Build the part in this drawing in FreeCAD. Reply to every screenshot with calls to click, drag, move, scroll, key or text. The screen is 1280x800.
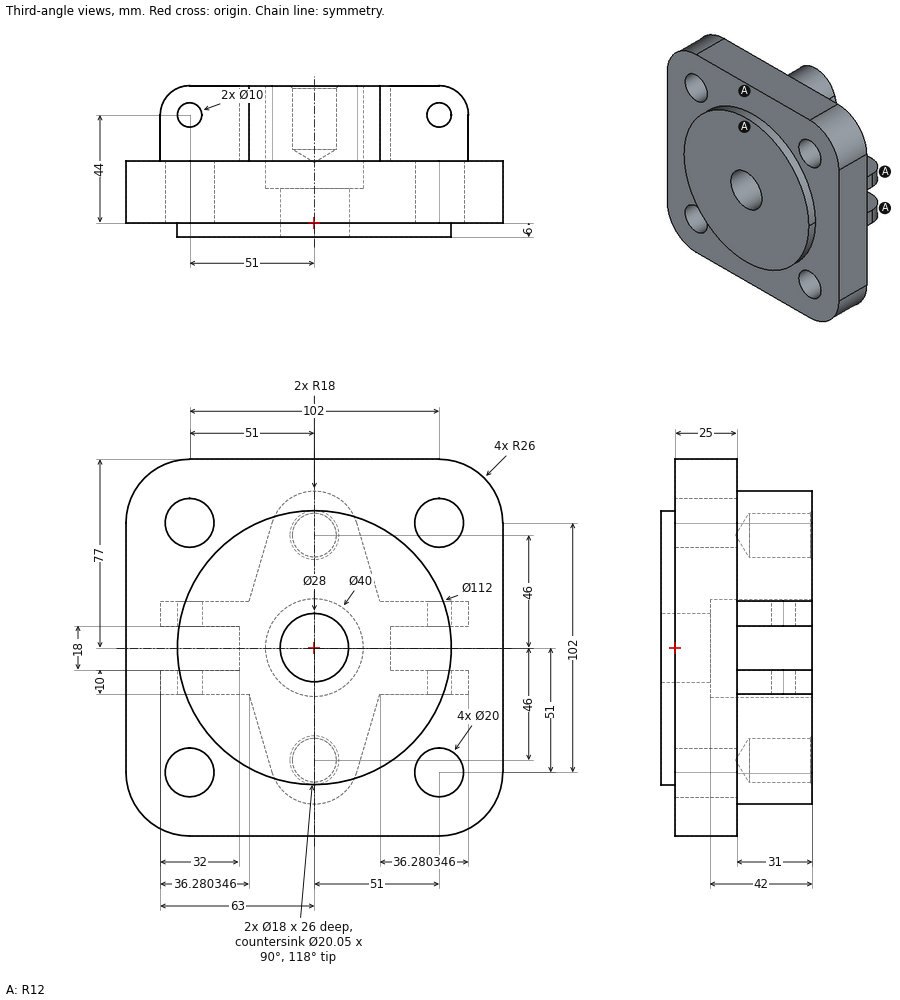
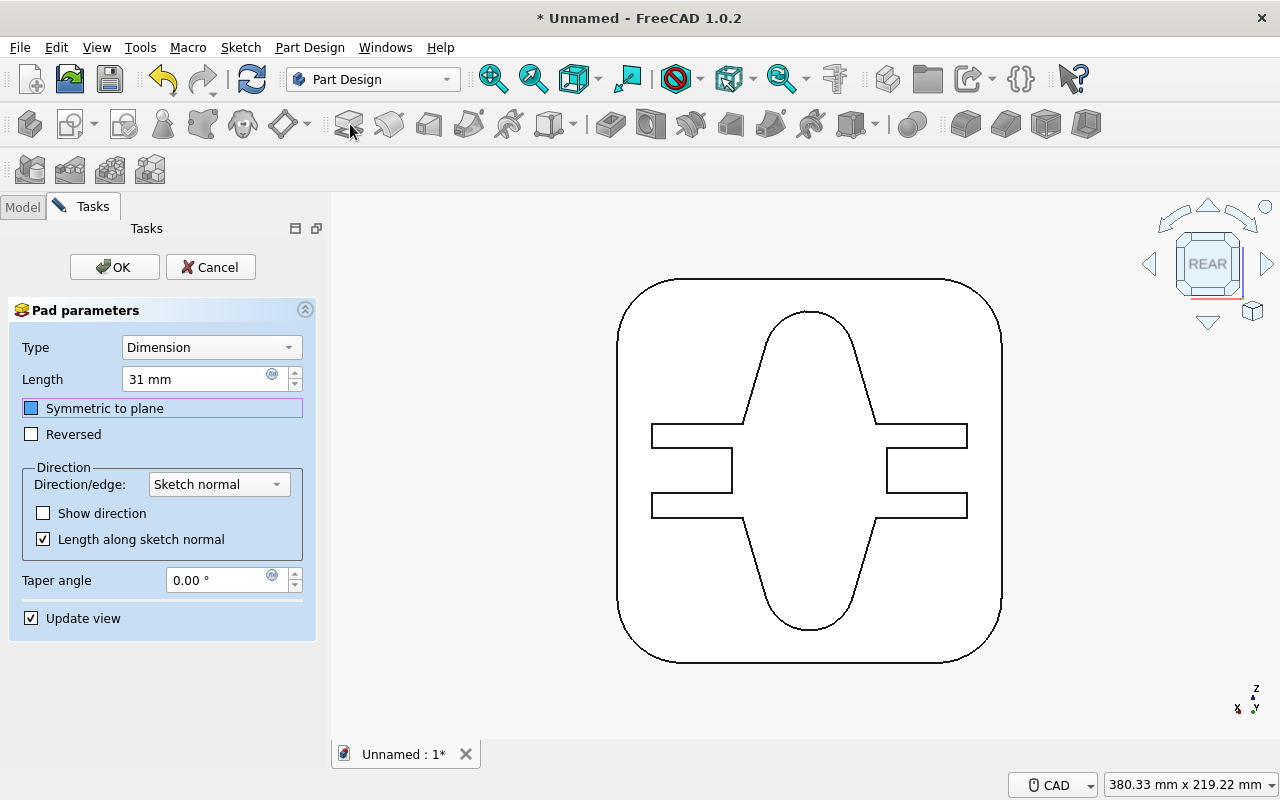
click(115, 267)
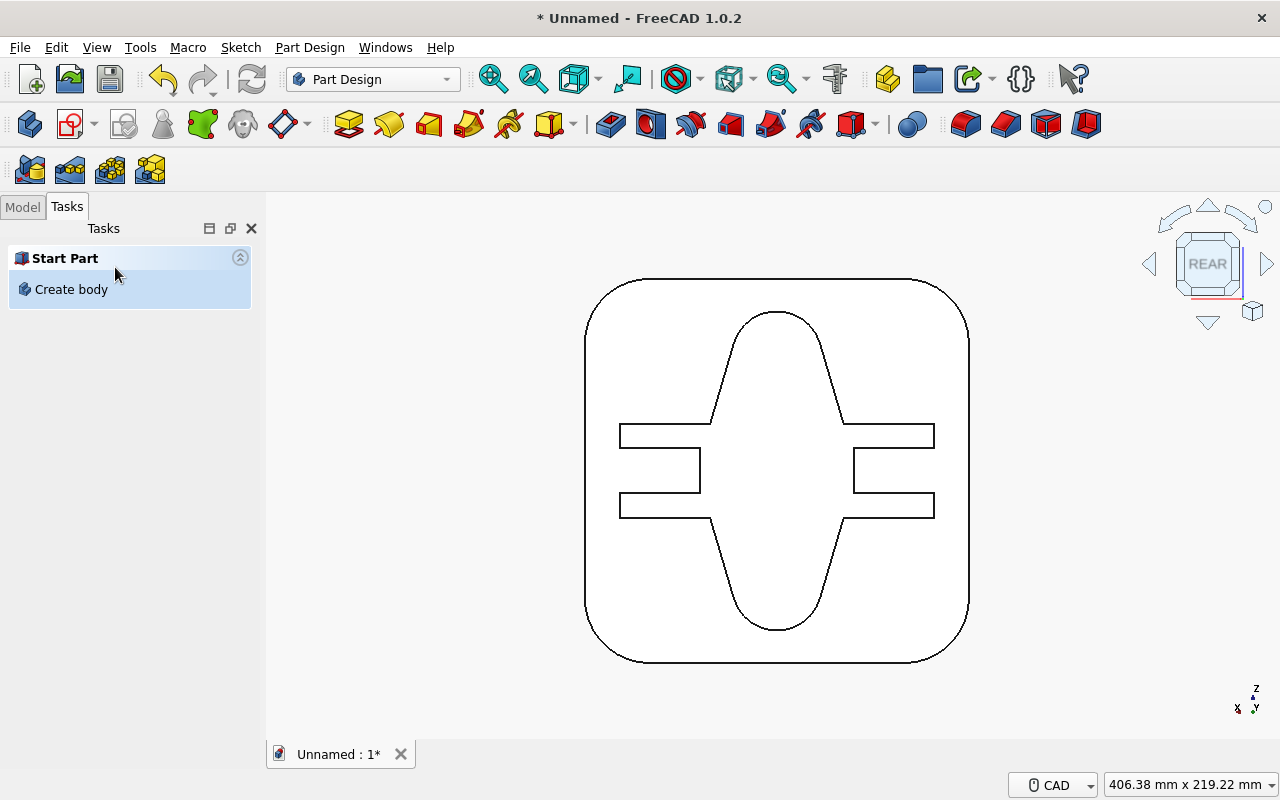
click(934, 435)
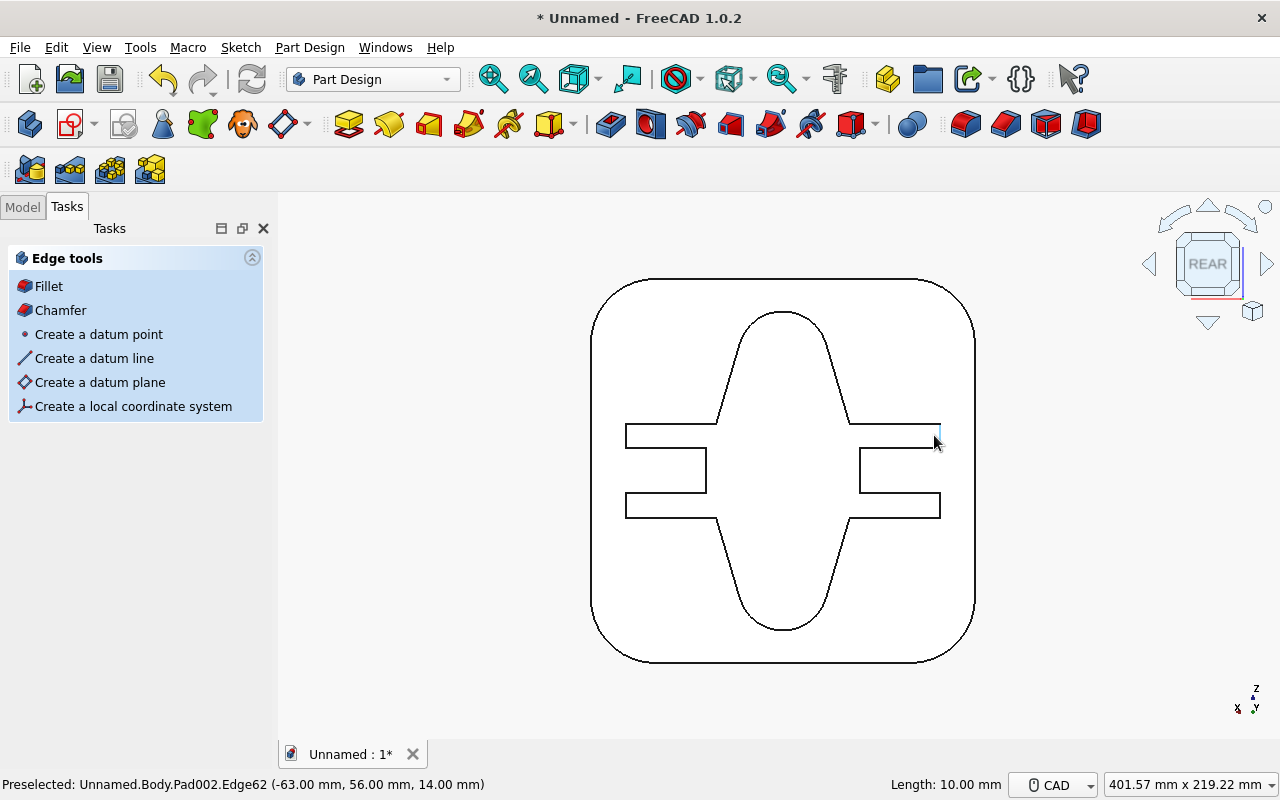
click(940, 505, ctrl)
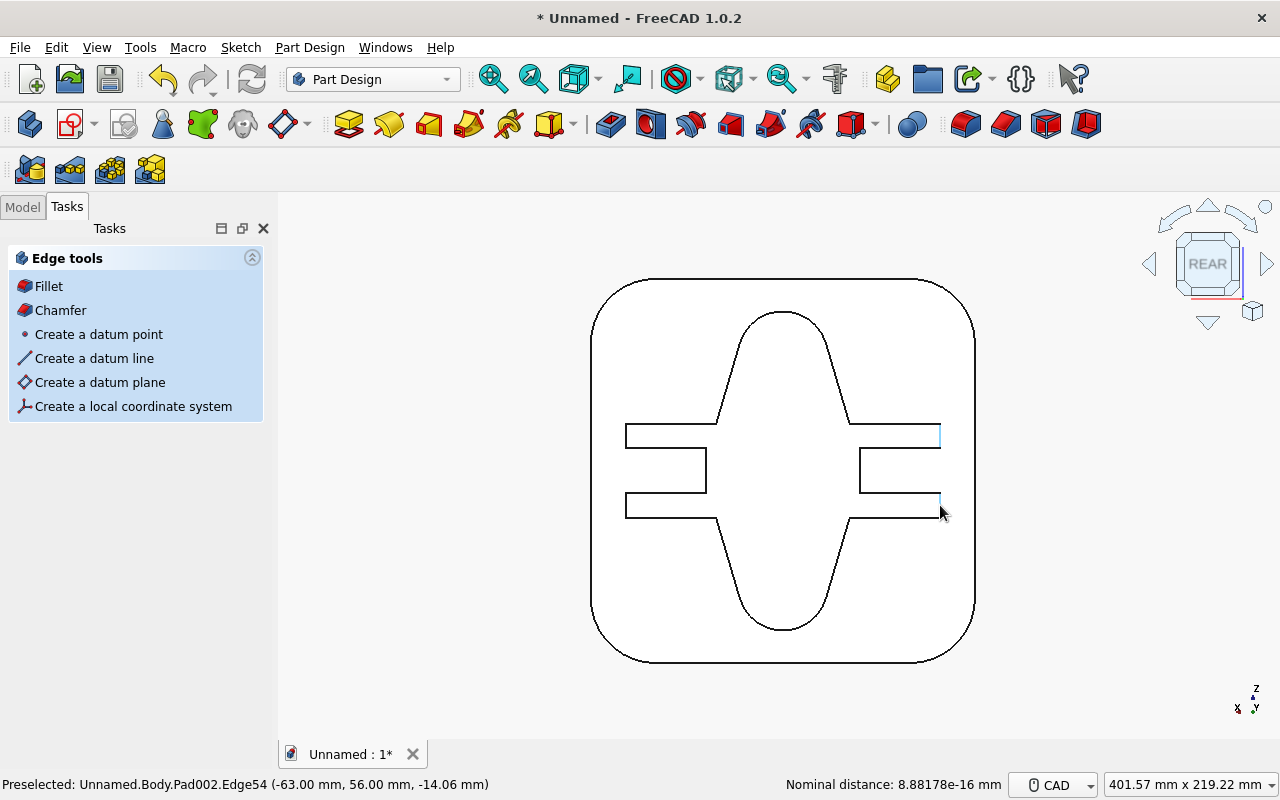
key(0)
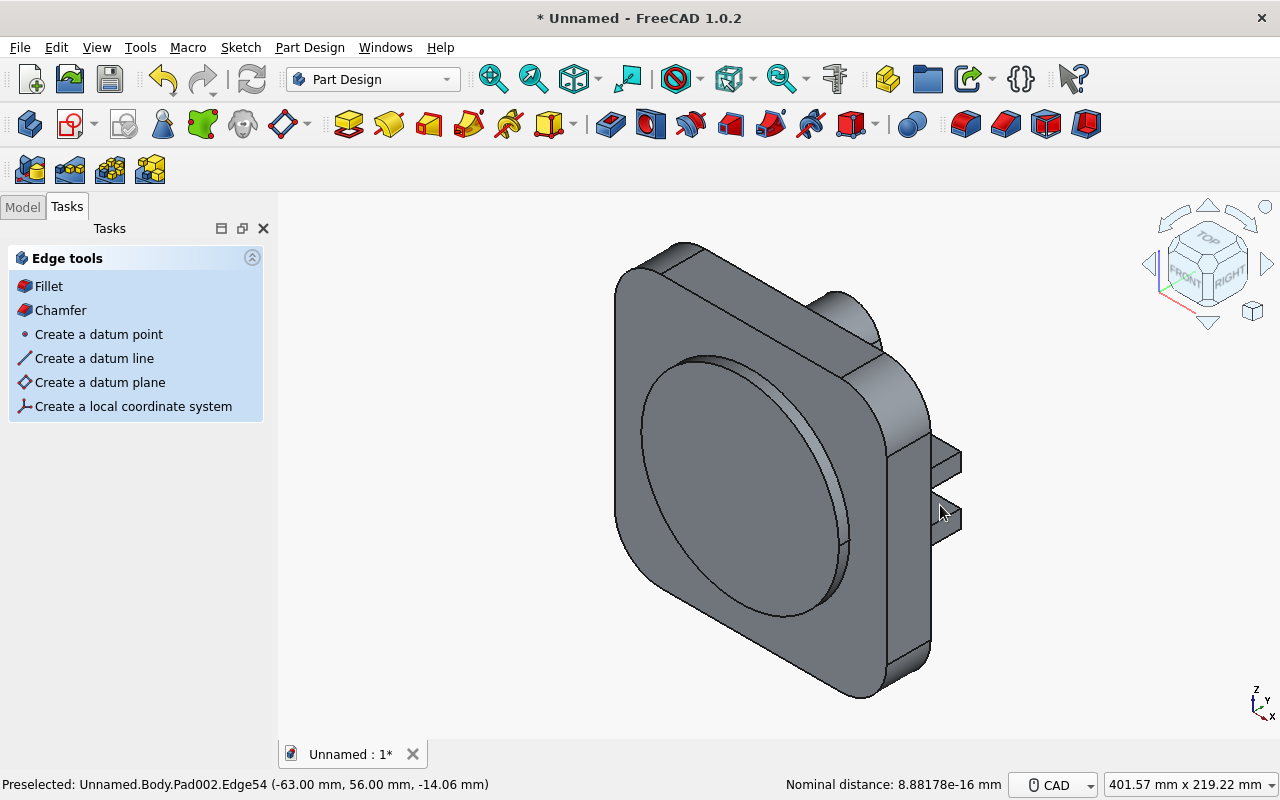
key(v)
key(f)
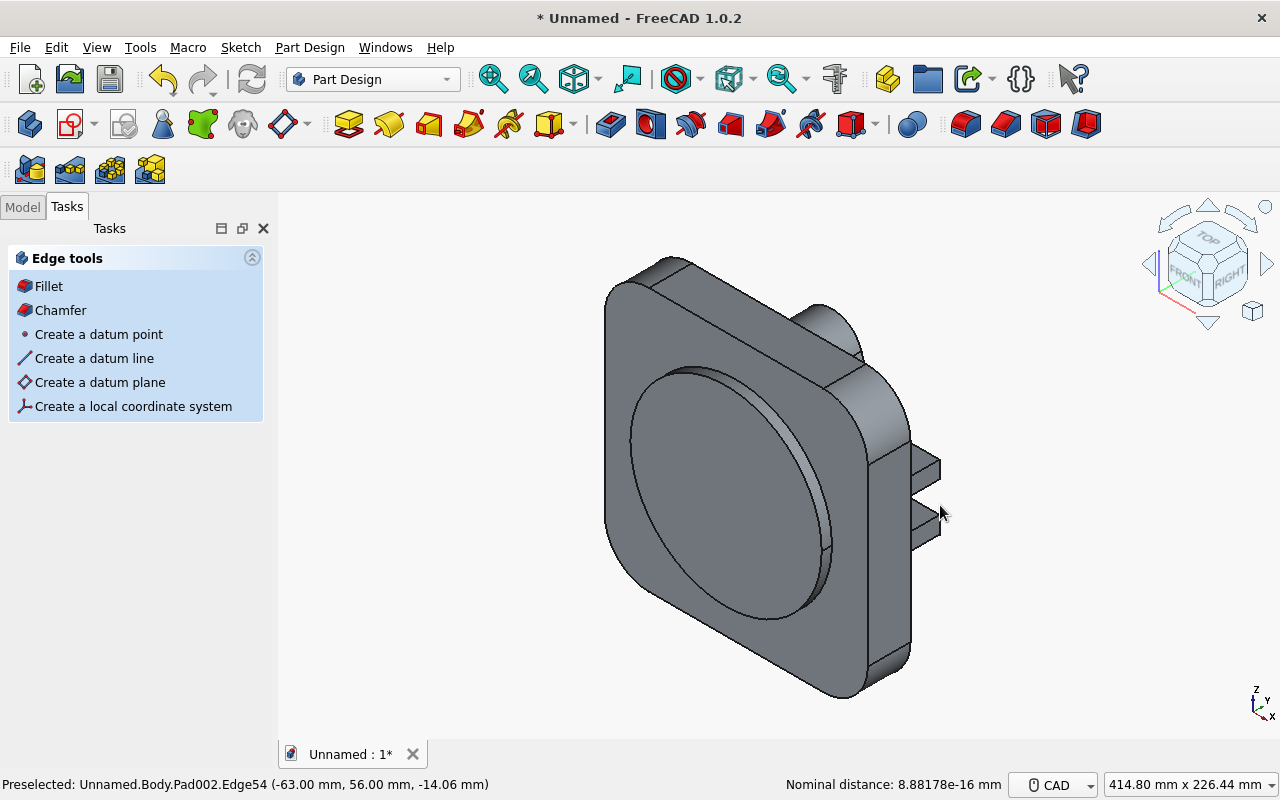
key(2)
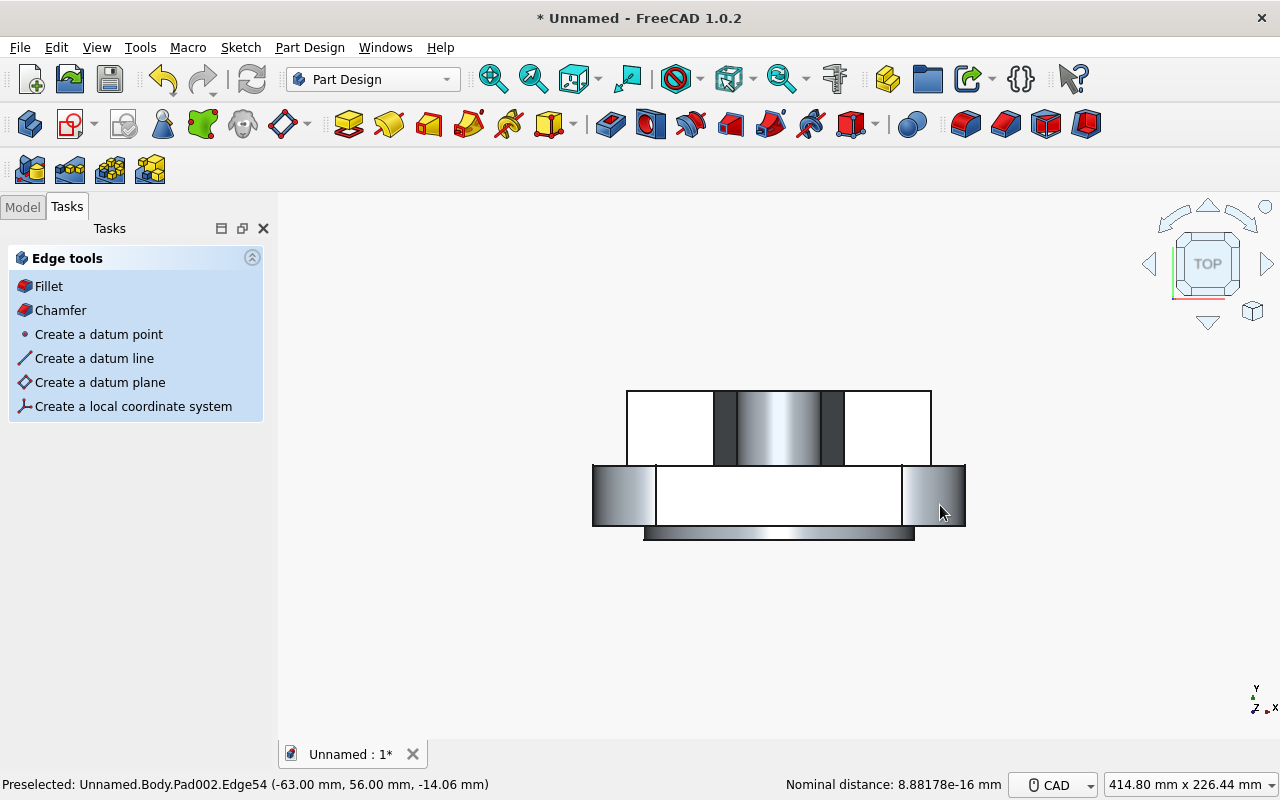
click(494, 80)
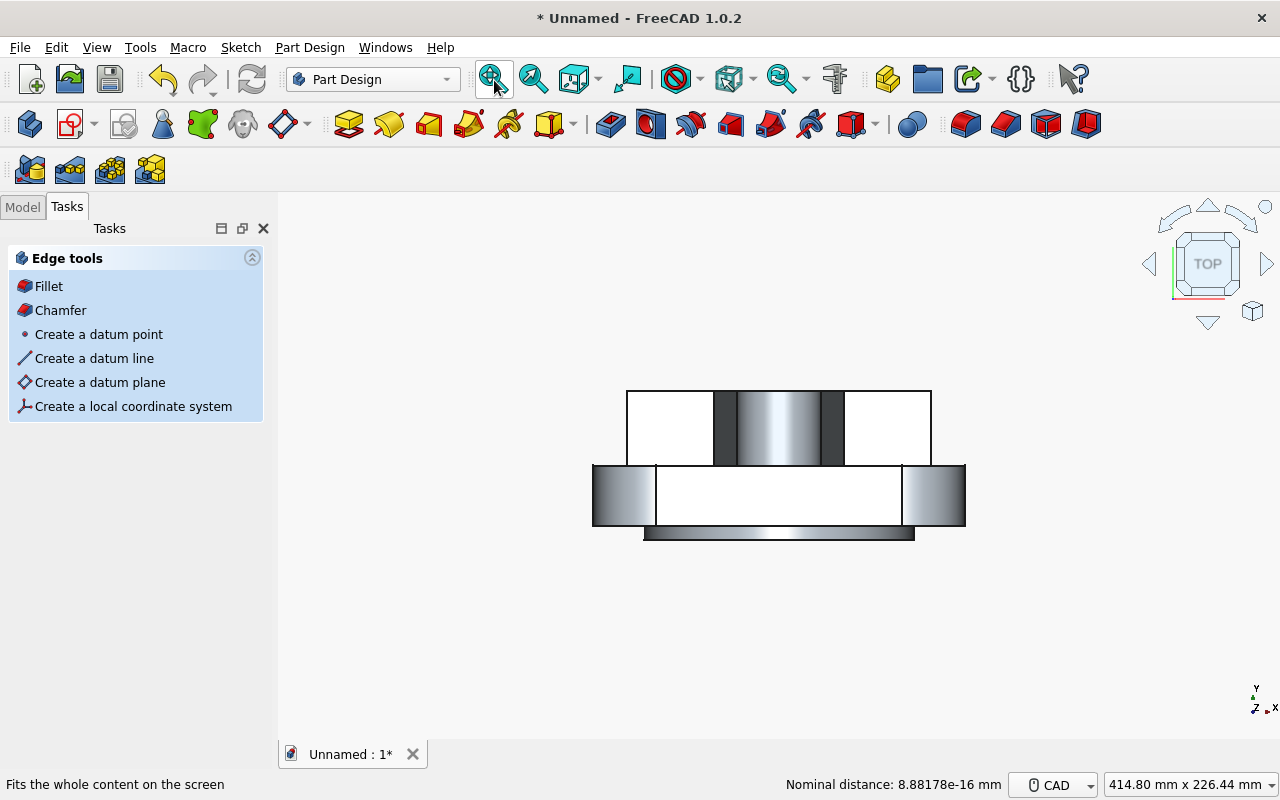
key(1)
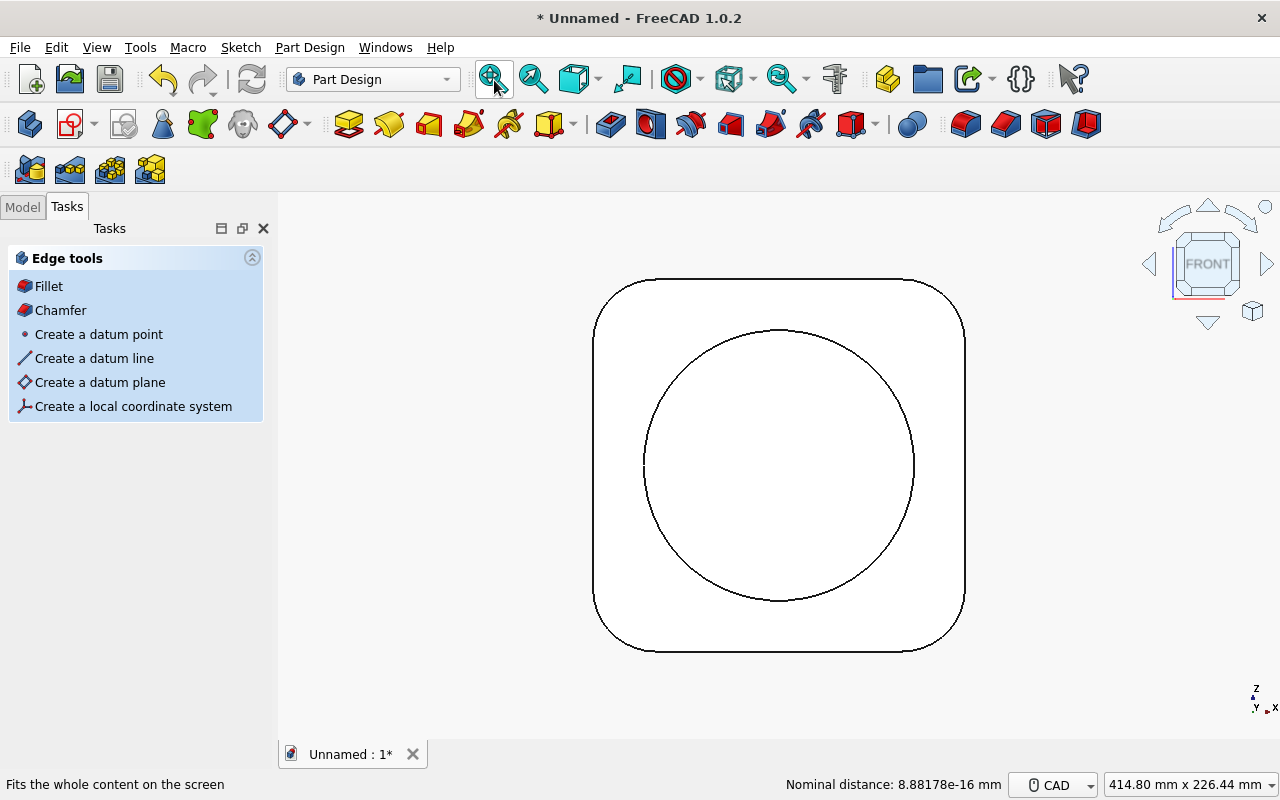
key(3)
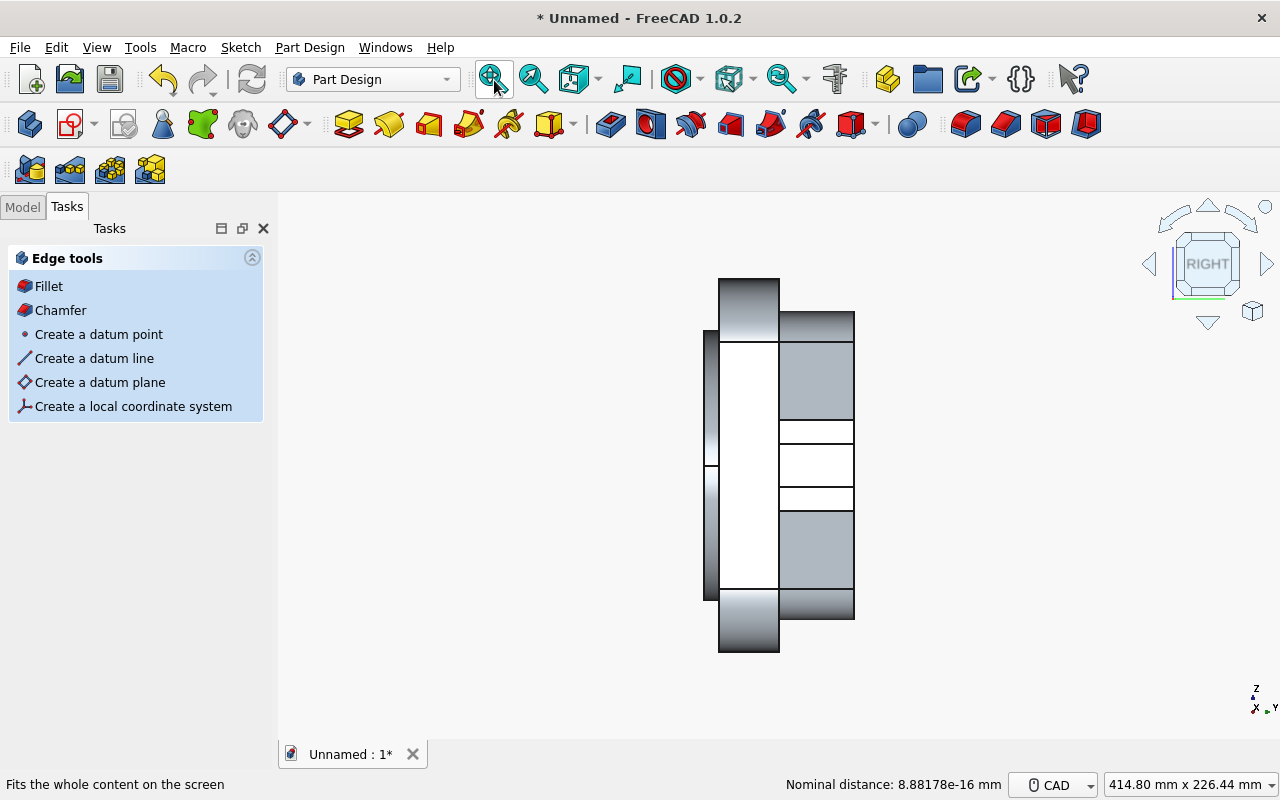
click(854, 431, ctrl)